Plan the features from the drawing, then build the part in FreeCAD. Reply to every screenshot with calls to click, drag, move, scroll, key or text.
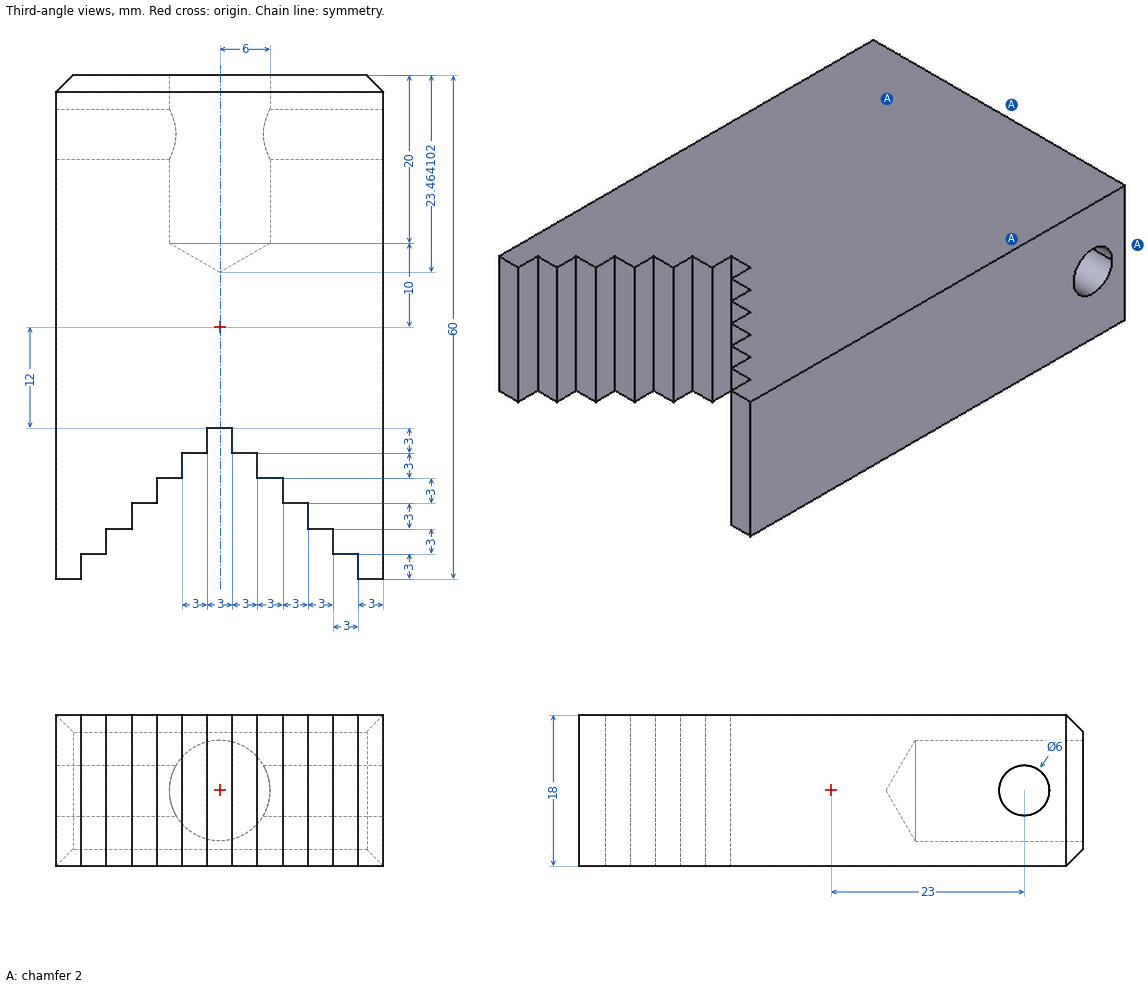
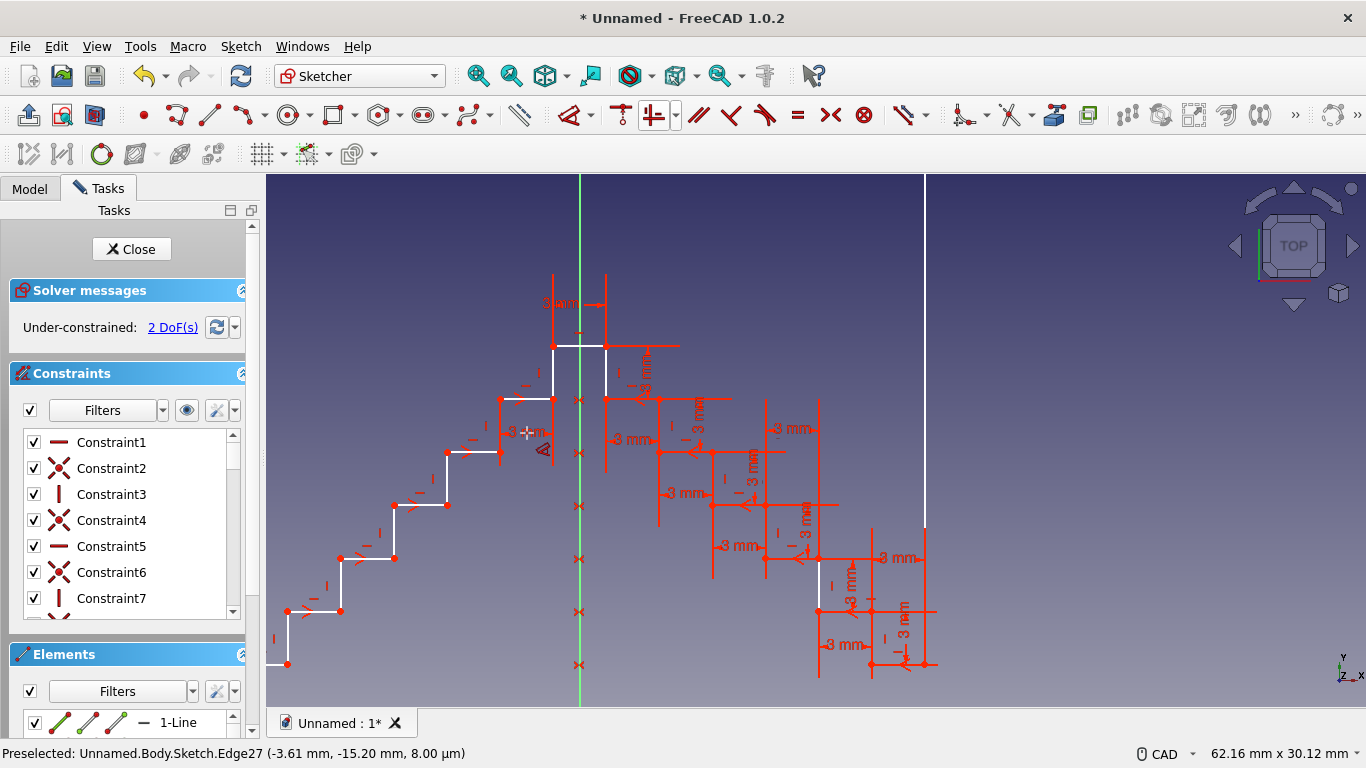
click(925, 346)
click(959, 433)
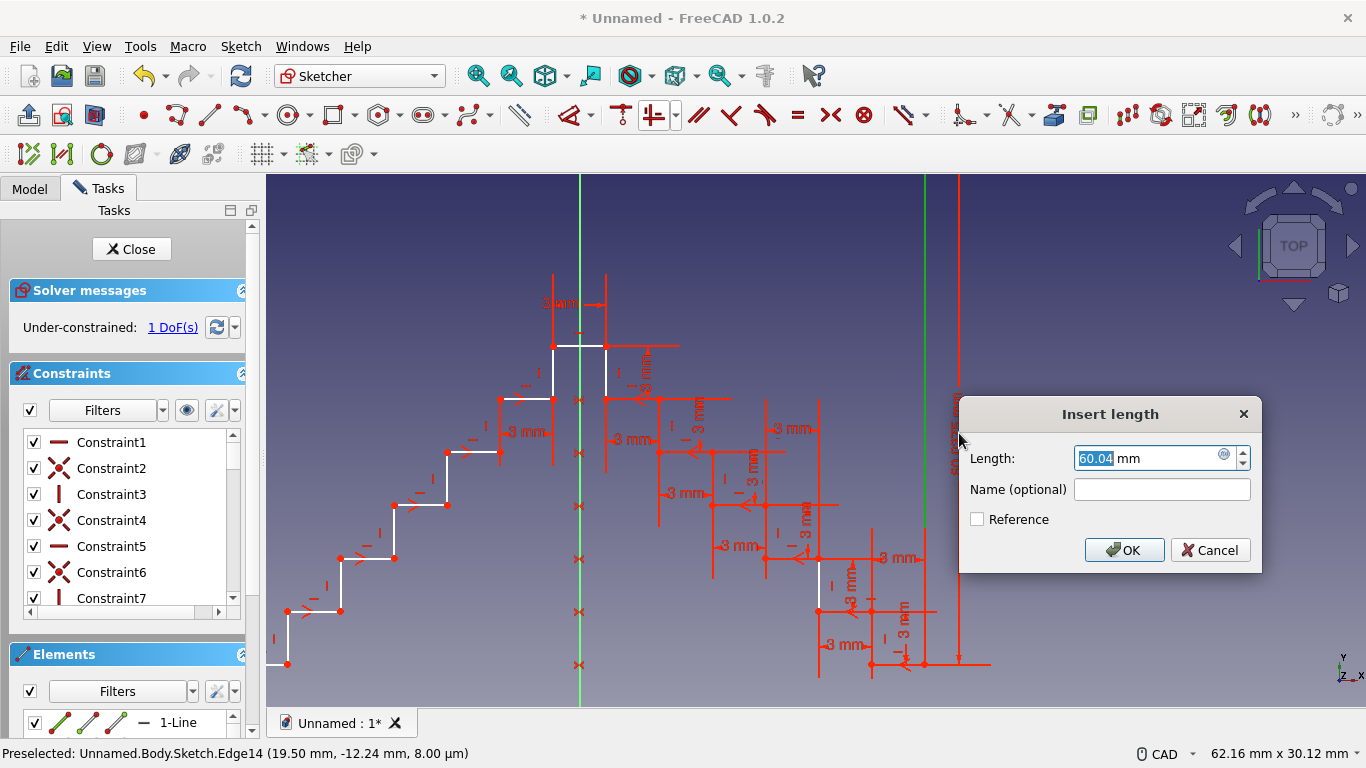
text(60)
key(Return)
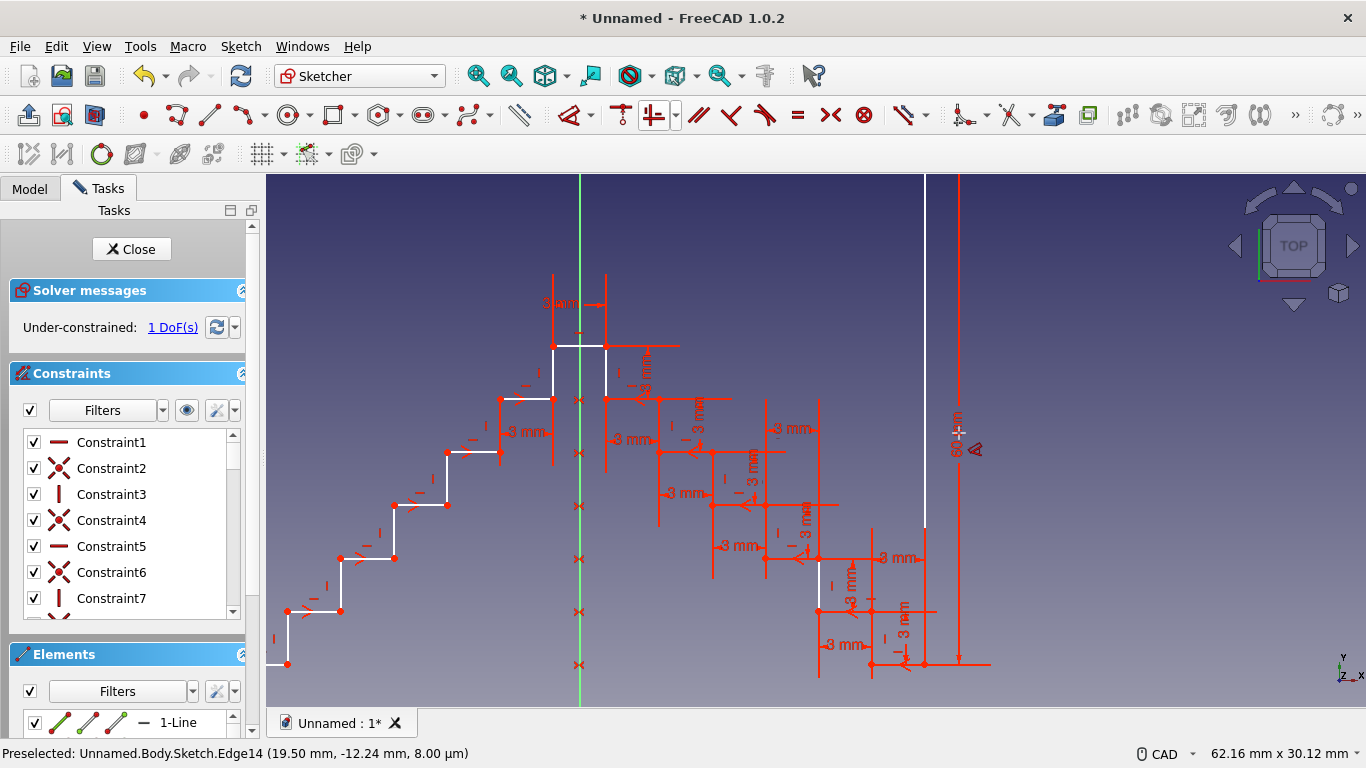
click(553, 346)
click(519, 274)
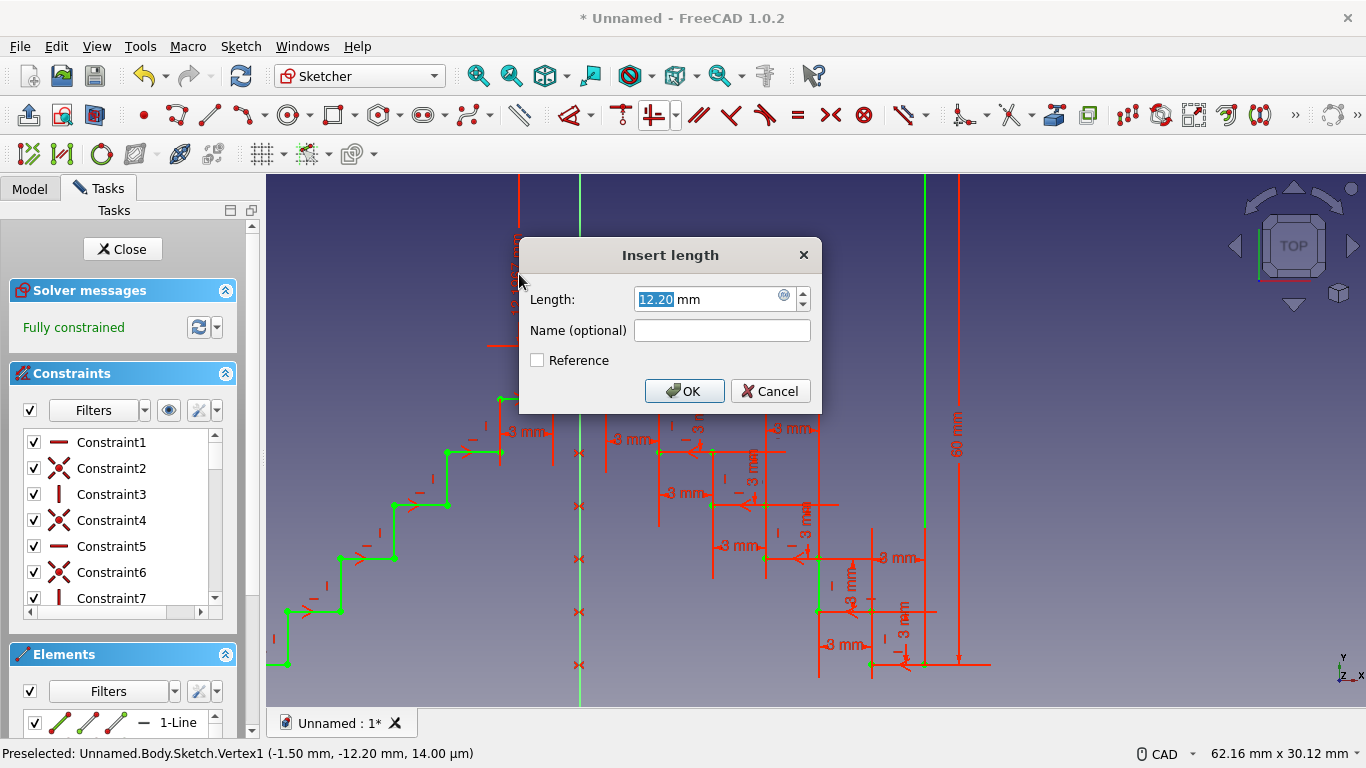
text(12)
key(Return)
key(Escape)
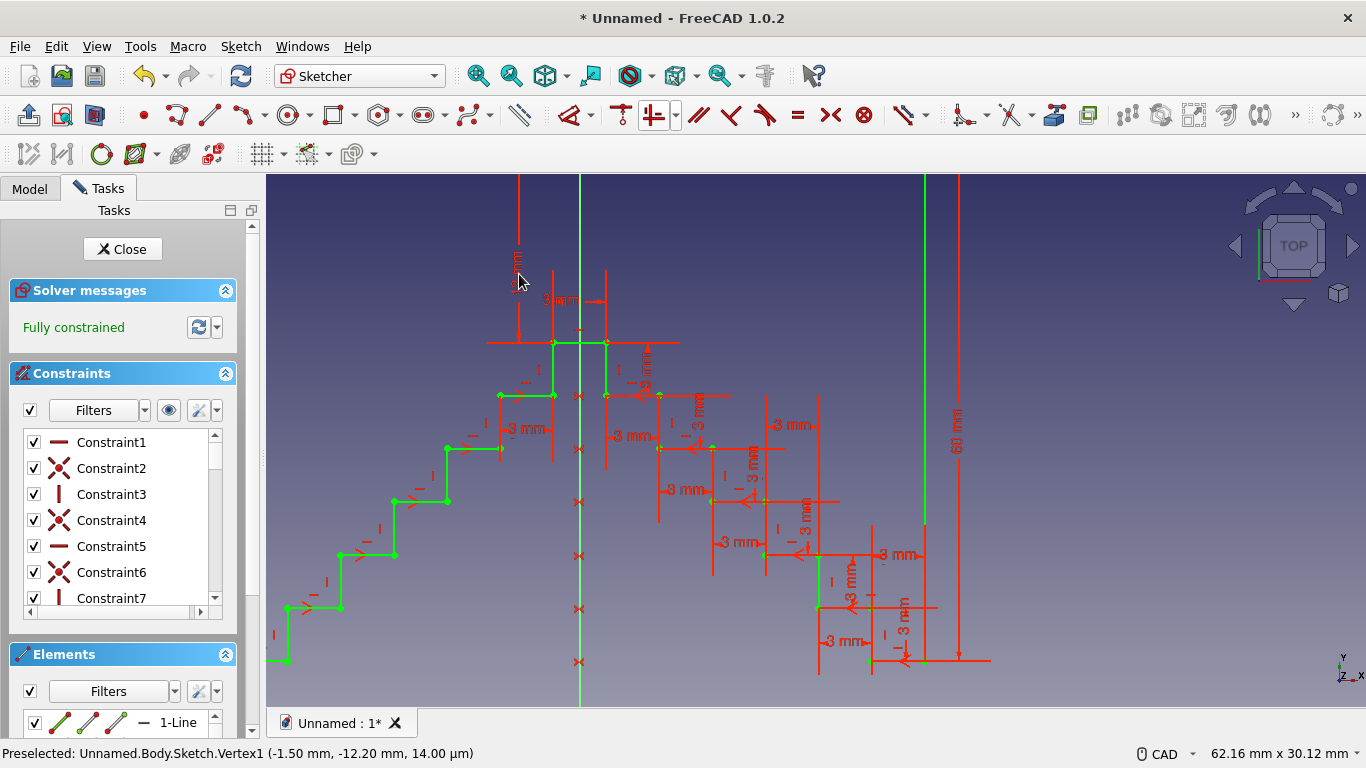
click(123, 249)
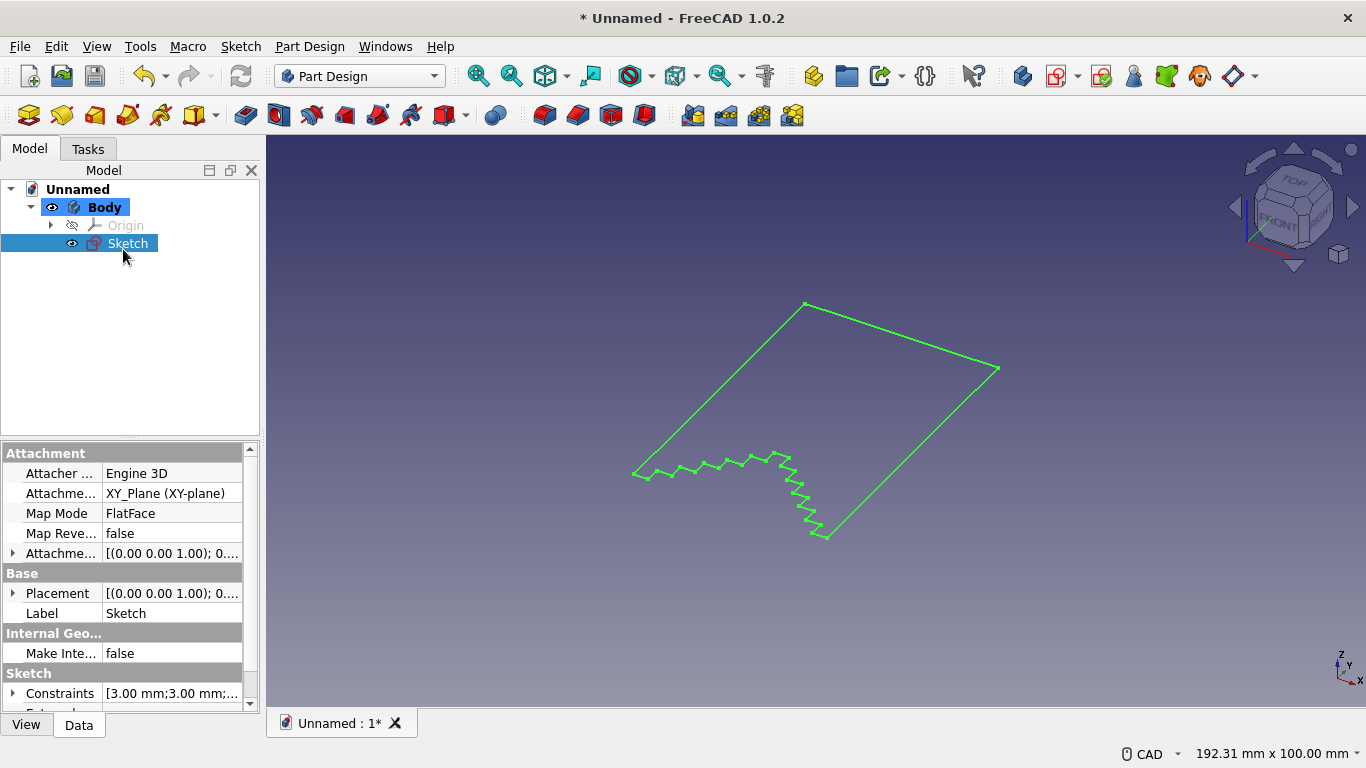
click(29, 116)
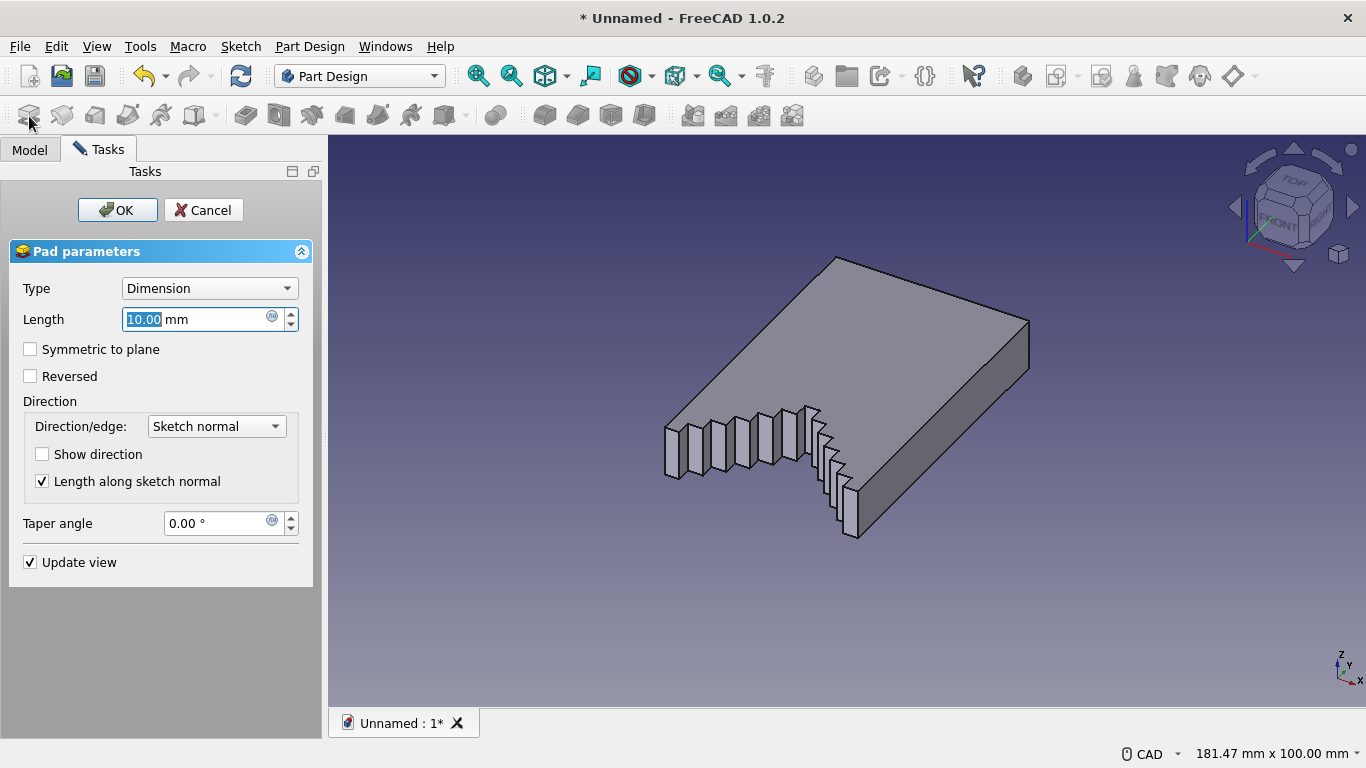
text(18)
key(Tab)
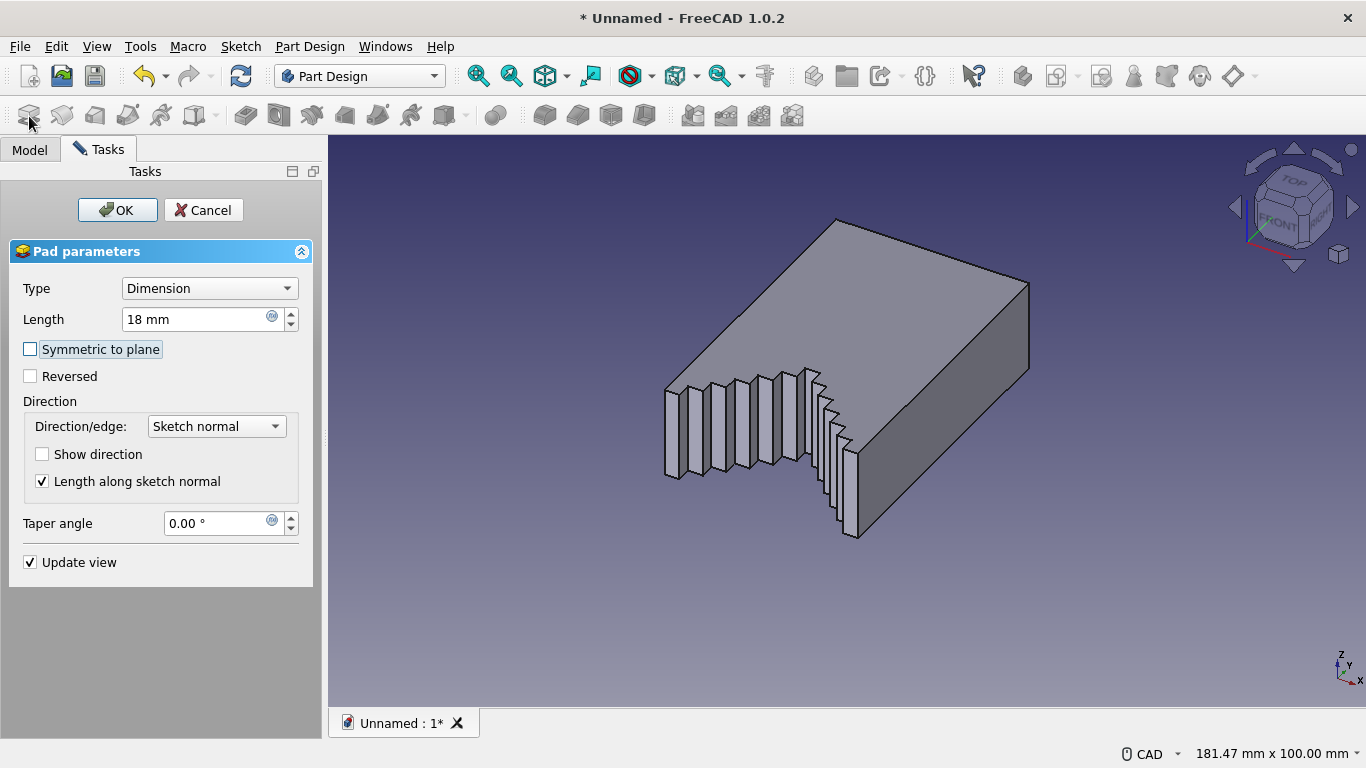
click(31, 349)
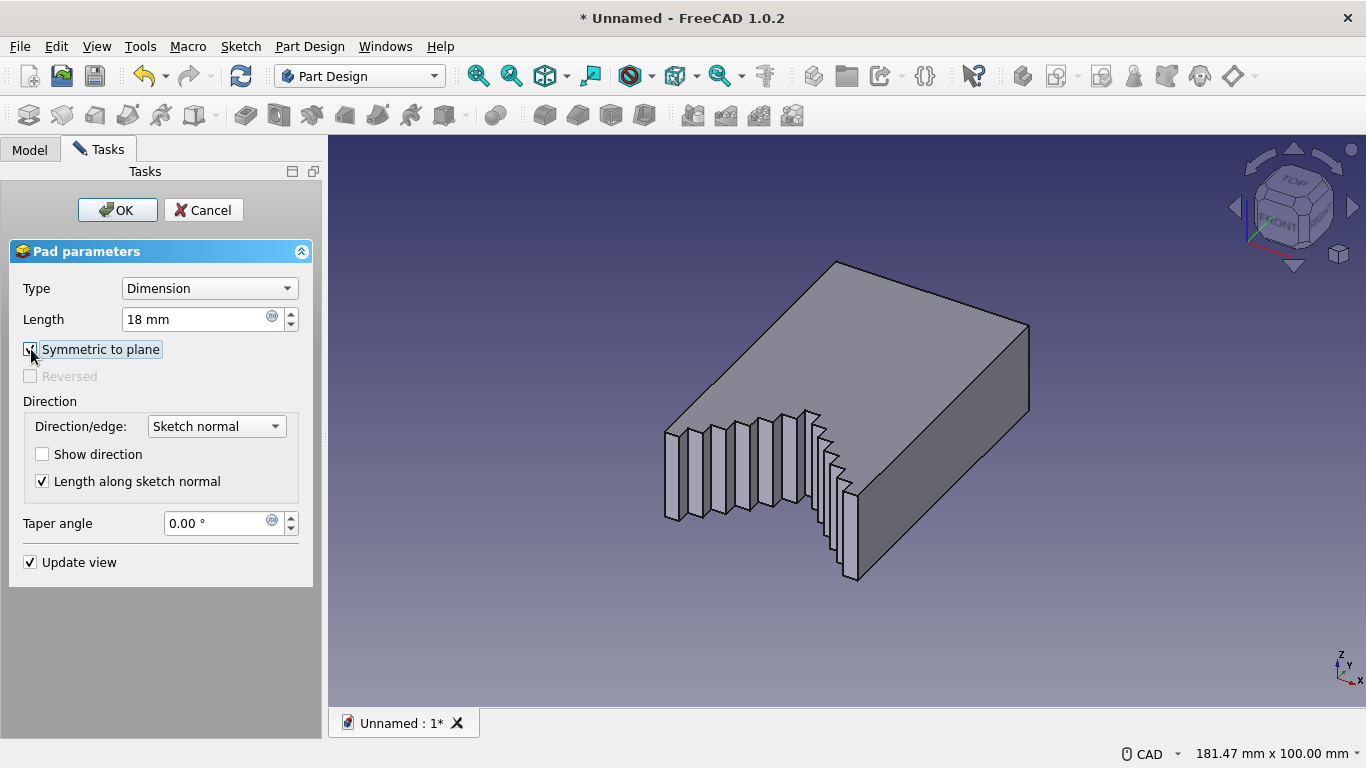
click(118, 210)